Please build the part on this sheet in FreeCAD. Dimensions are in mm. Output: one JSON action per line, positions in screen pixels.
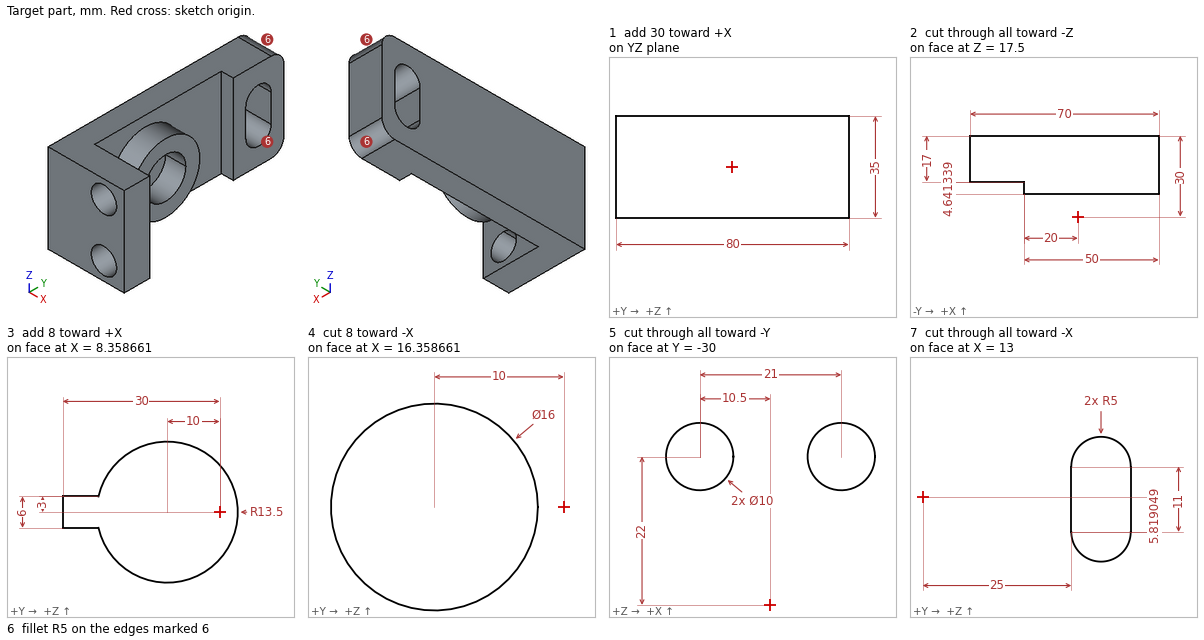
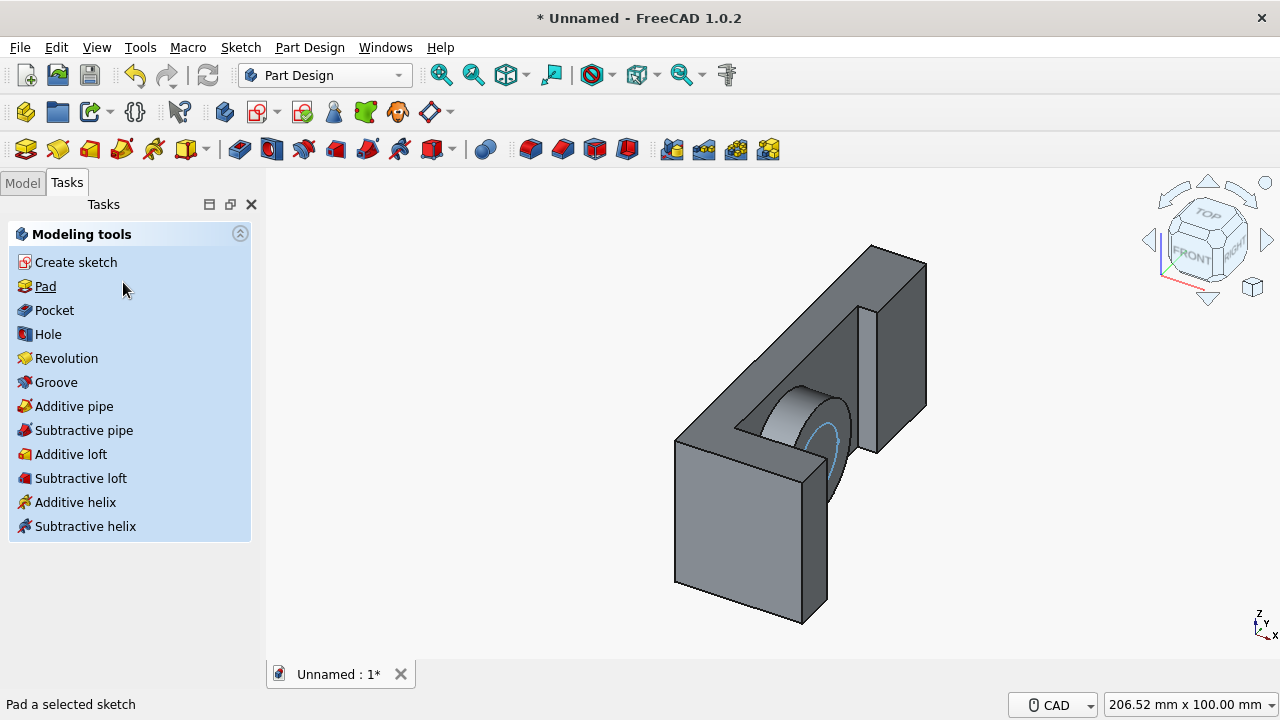
{"action": "left_click", "coordinate": [240, 150]}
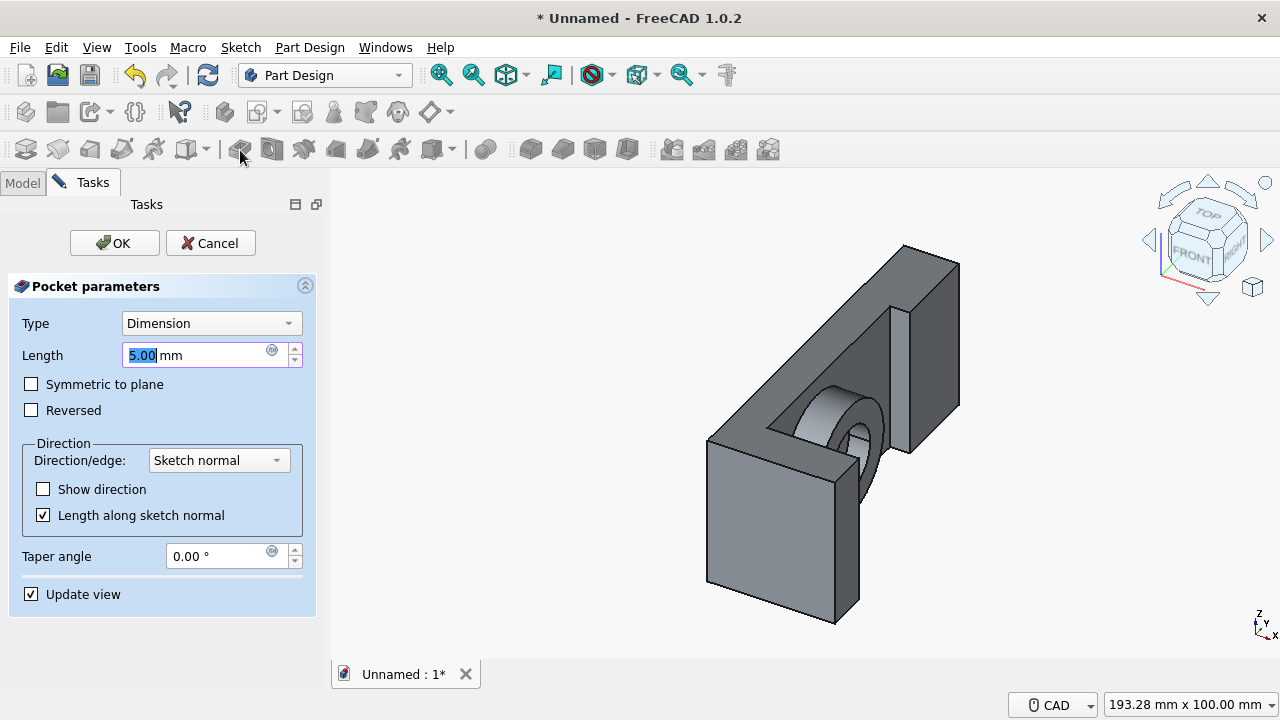
{"action": "type", "text": "8"}
{"action": "key", "text": "Tab"}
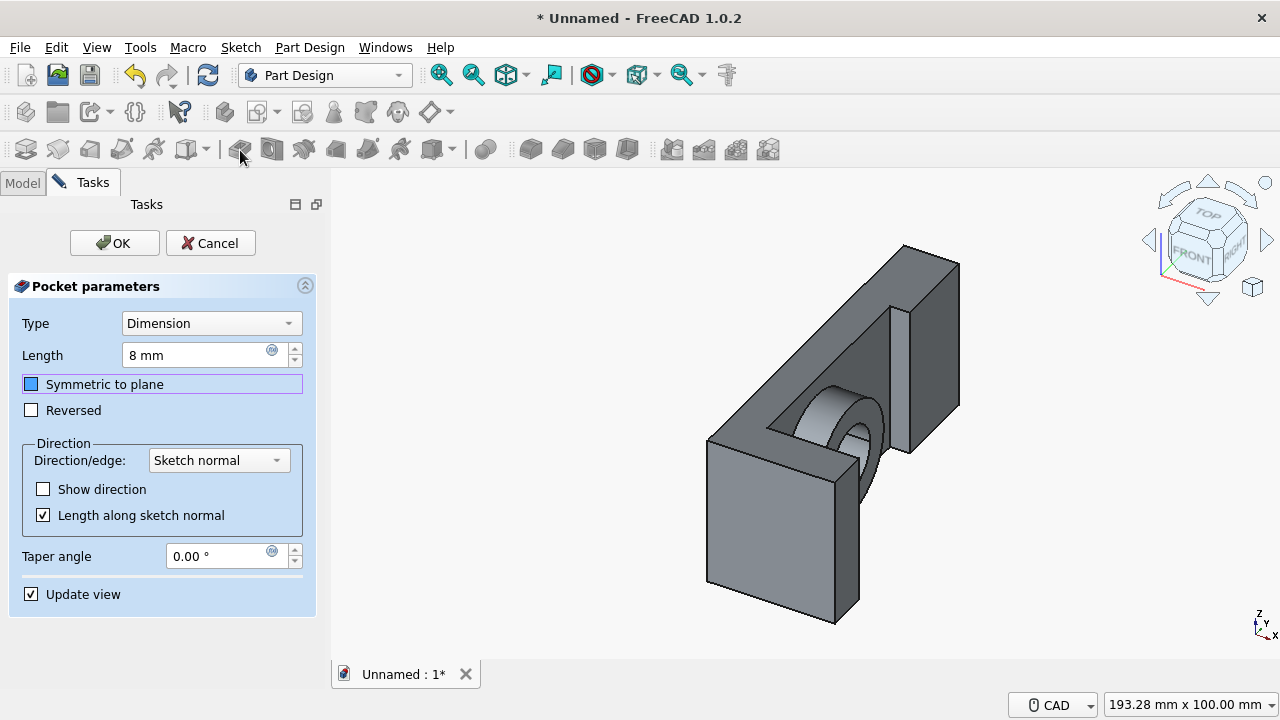
{"action": "left_click", "coordinate": [115, 243]}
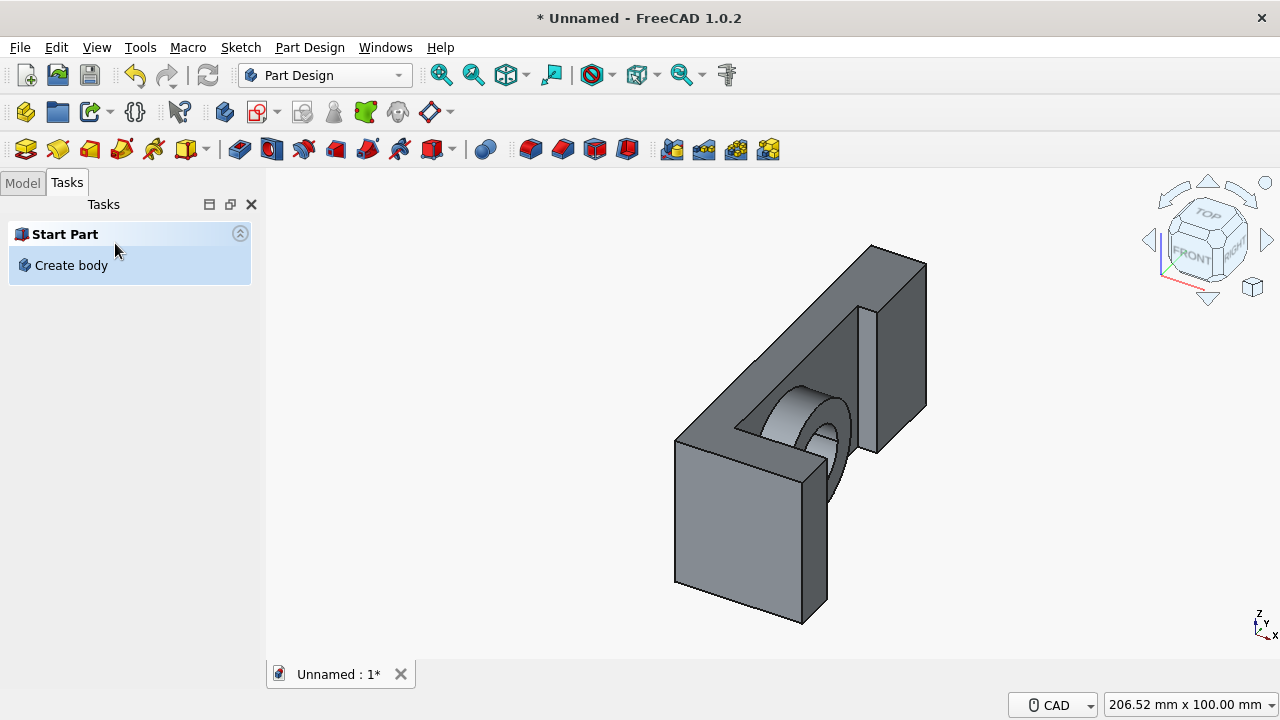
{"action": "key", "text": "4"}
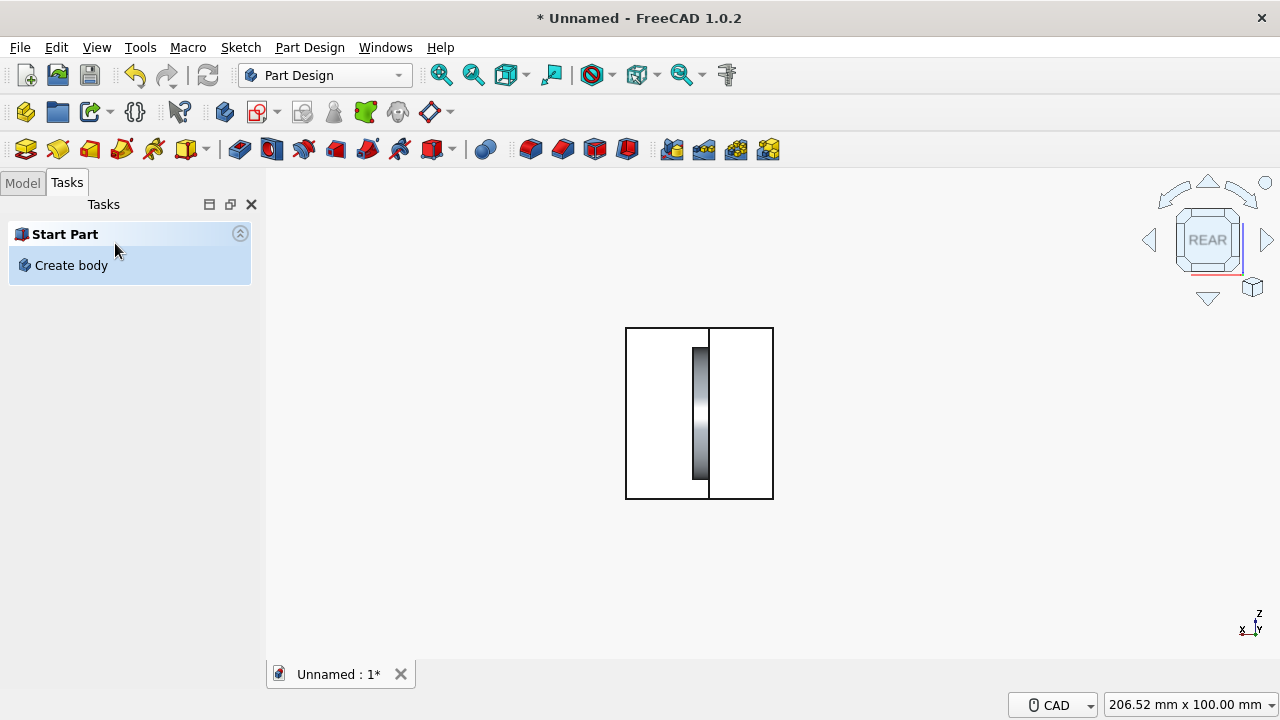
{"action": "key", "text": "v f"}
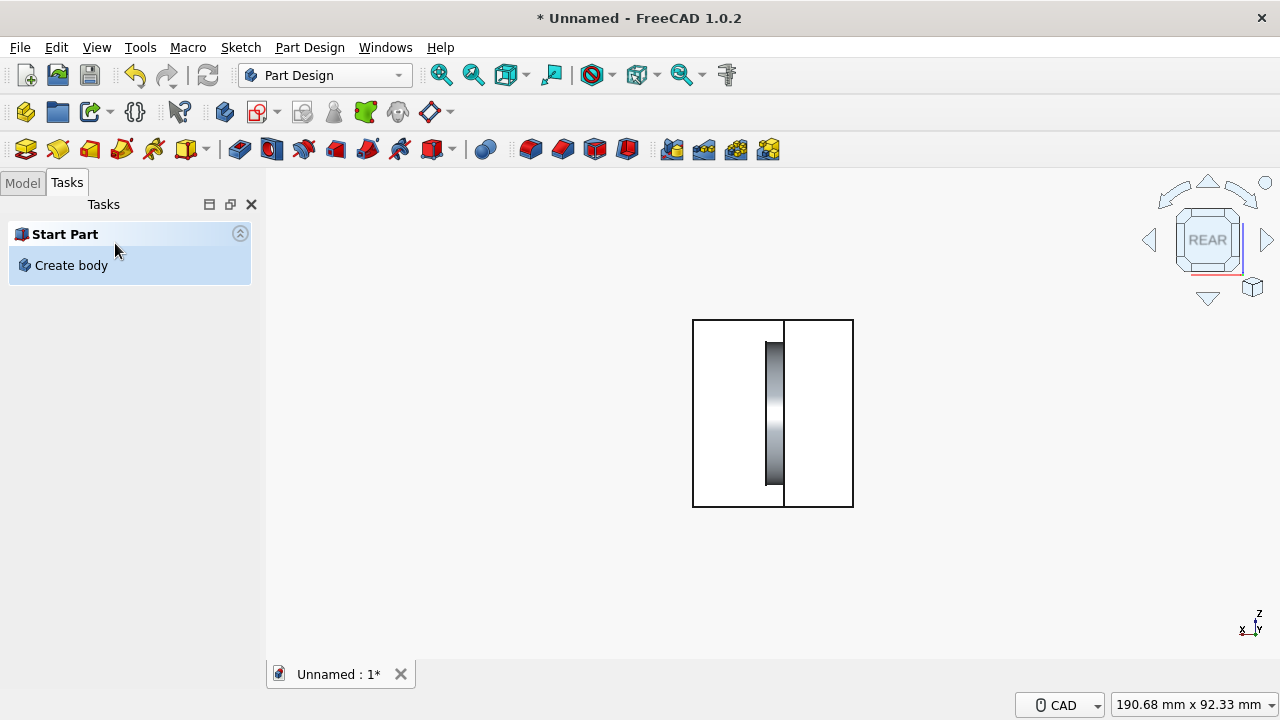
{"action": "left_click", "coordinate": [734, 359]}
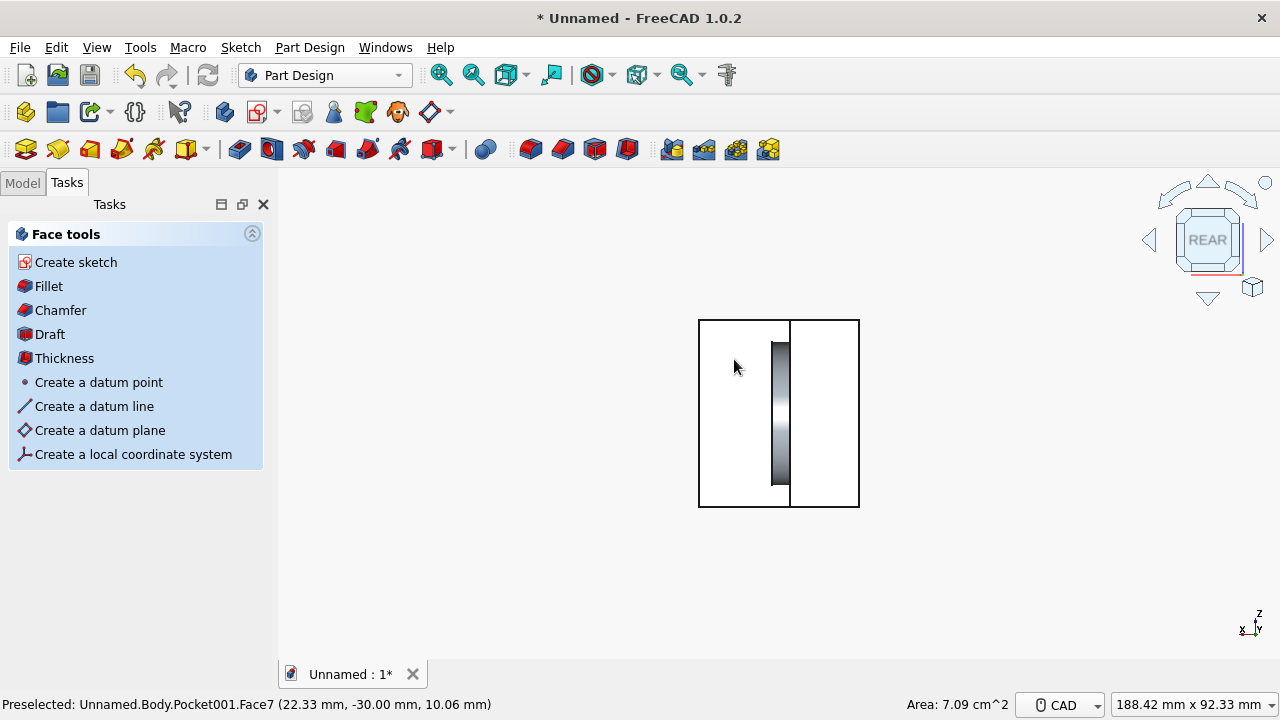
{"action": "left_click", "coordinate": [258, 112]}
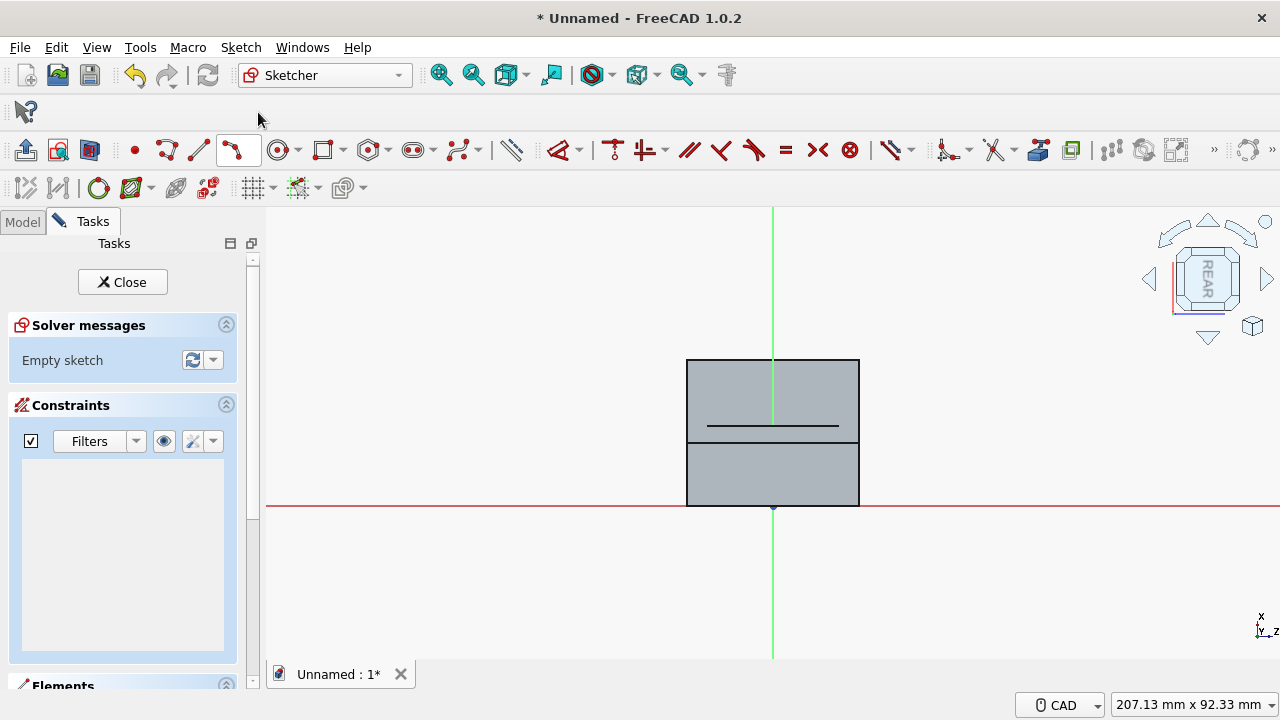
{"action": "scroll", "coordinate": [829, 446], "scroll_direction": "up", "scroll_amount": 4}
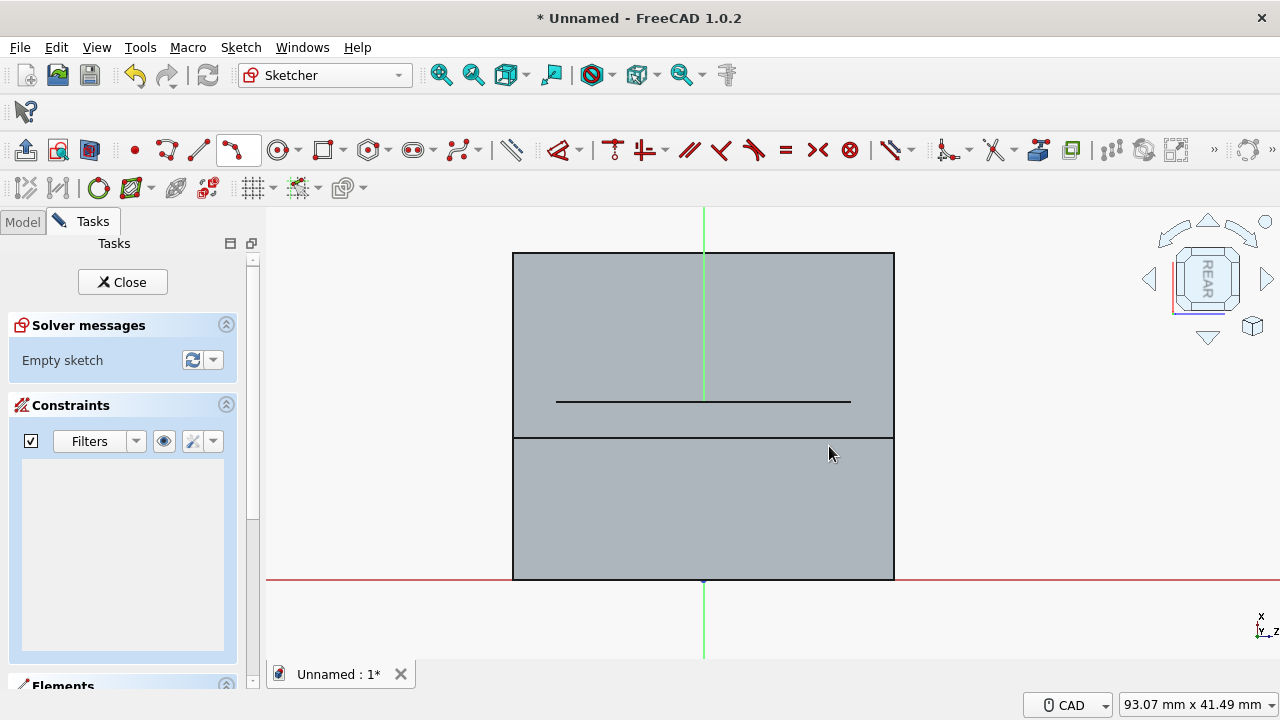
{"action": "left_click", "coordinate": [278, 150]}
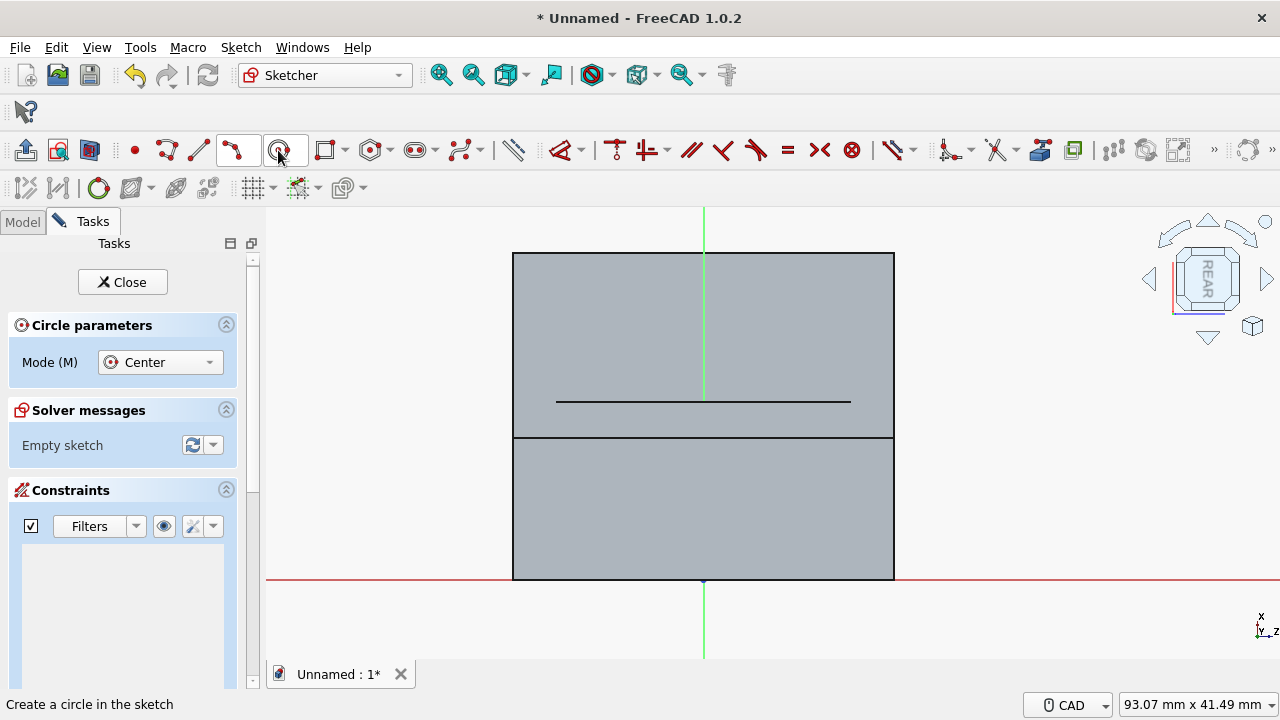
{"action": "left_click", "coordinate": [589, 340]}
{"action": "left_click", "coordinate": [628, 302]}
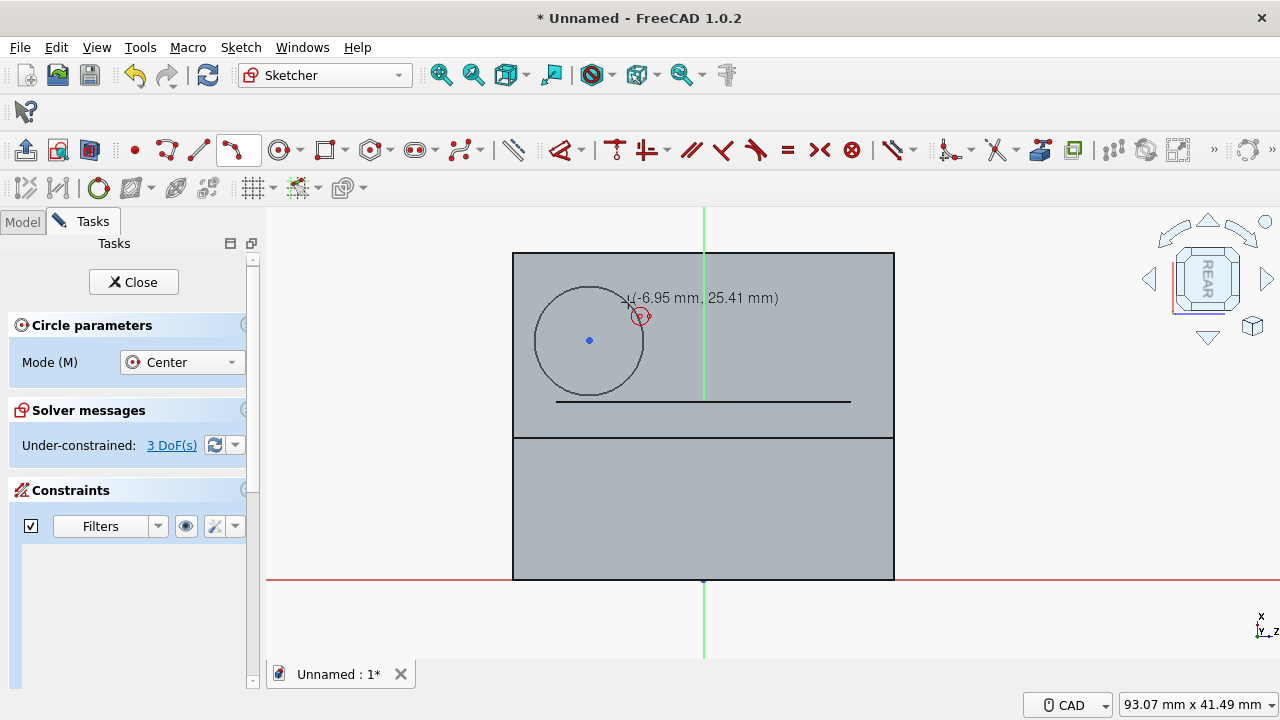
{"action": "left_click", "coordinate": [818, 340]}
{"action": "left_click", "coordinate": [857, 302]}
{"action": "key", "text": "Escape"}